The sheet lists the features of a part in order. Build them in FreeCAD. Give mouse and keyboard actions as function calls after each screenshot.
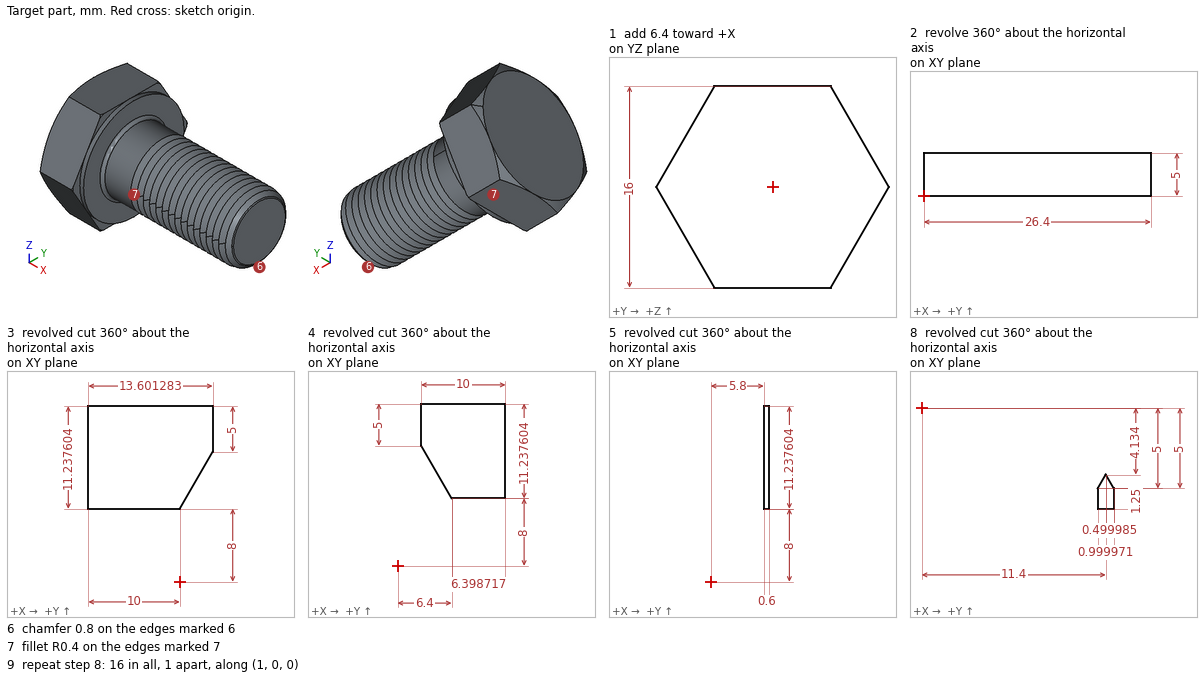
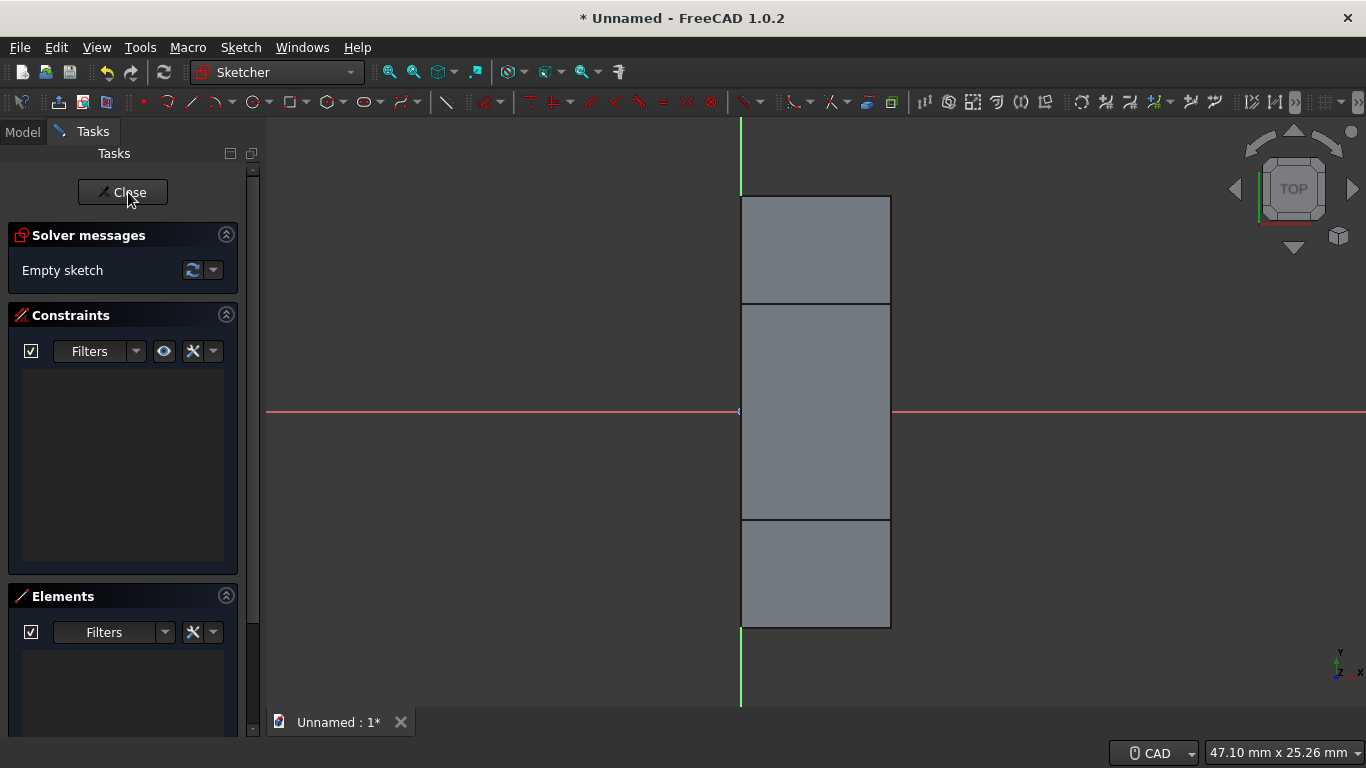
key(q)
key(s)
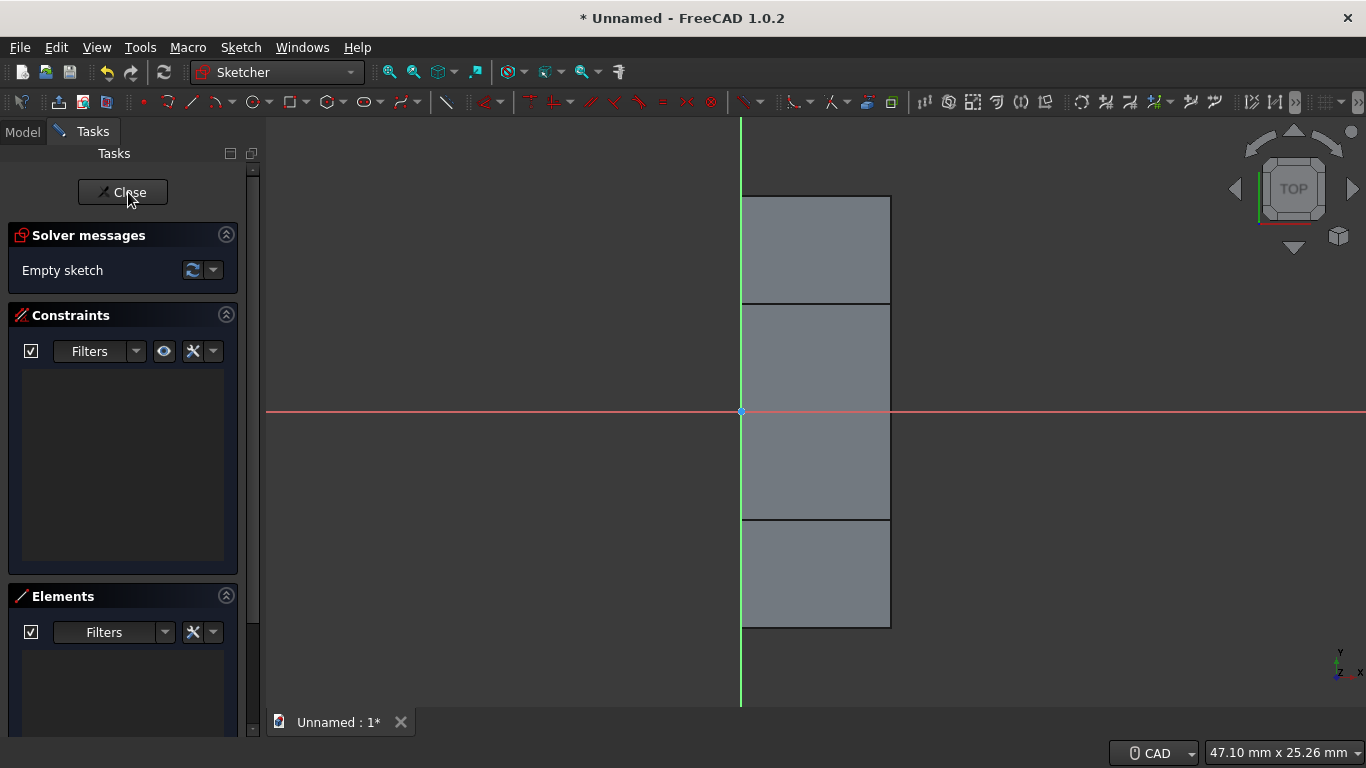
scroll(294, 676, down, 1)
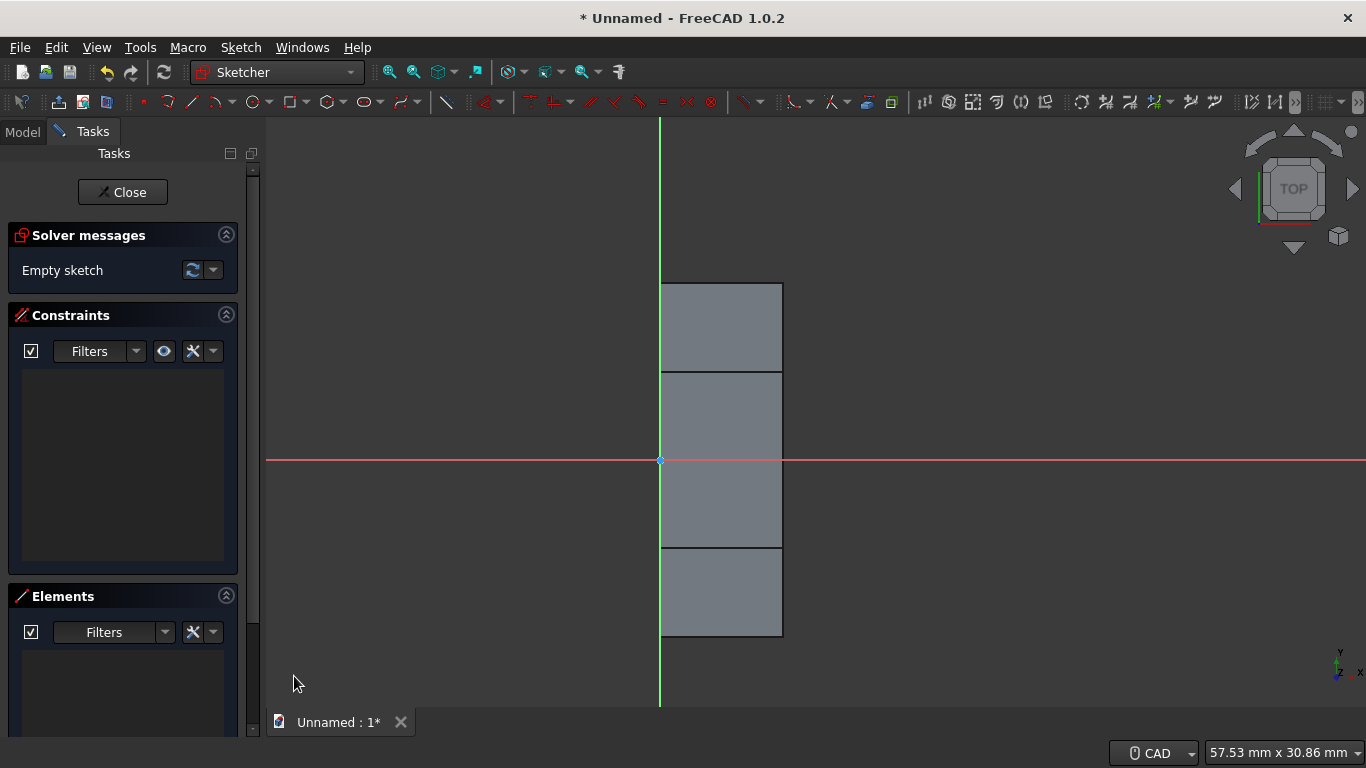
key(g)
key(r)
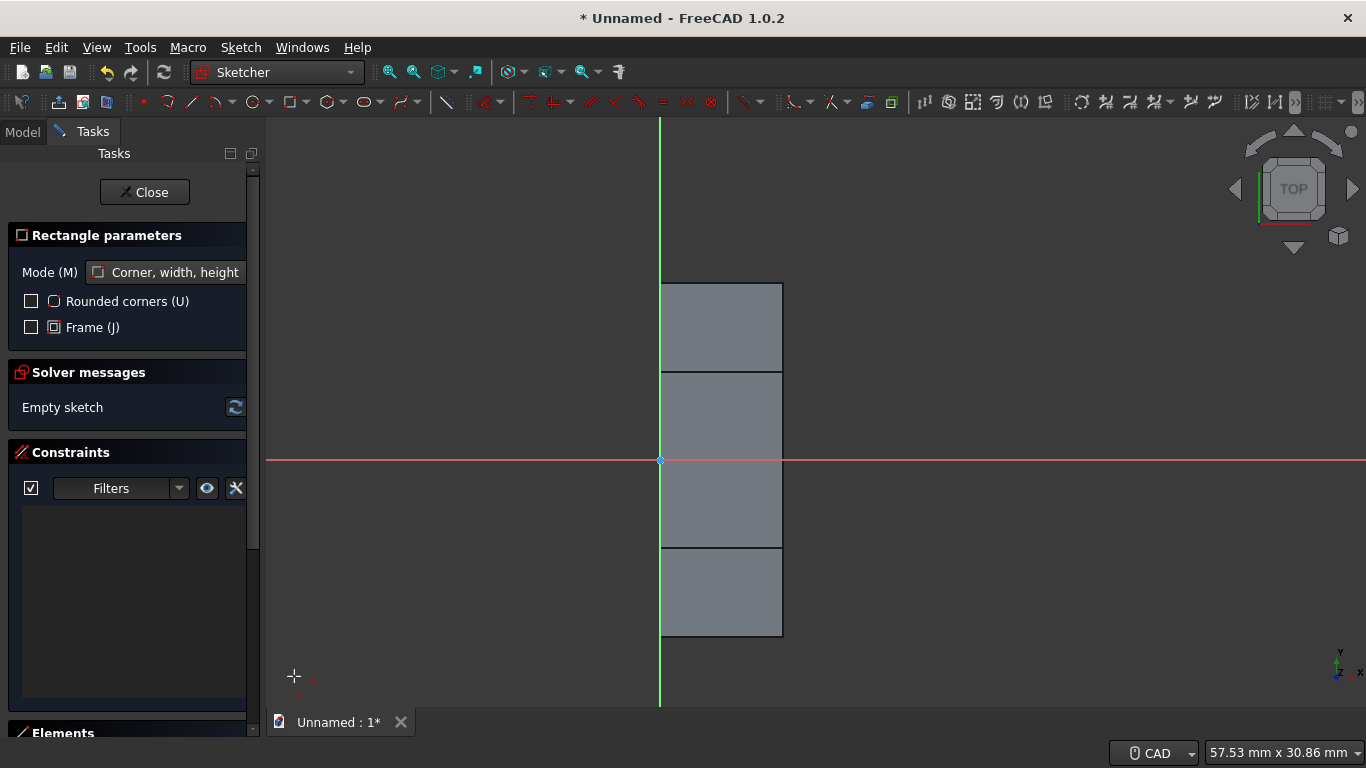
click(660, 460)
click(1165, 364)
key(Escape)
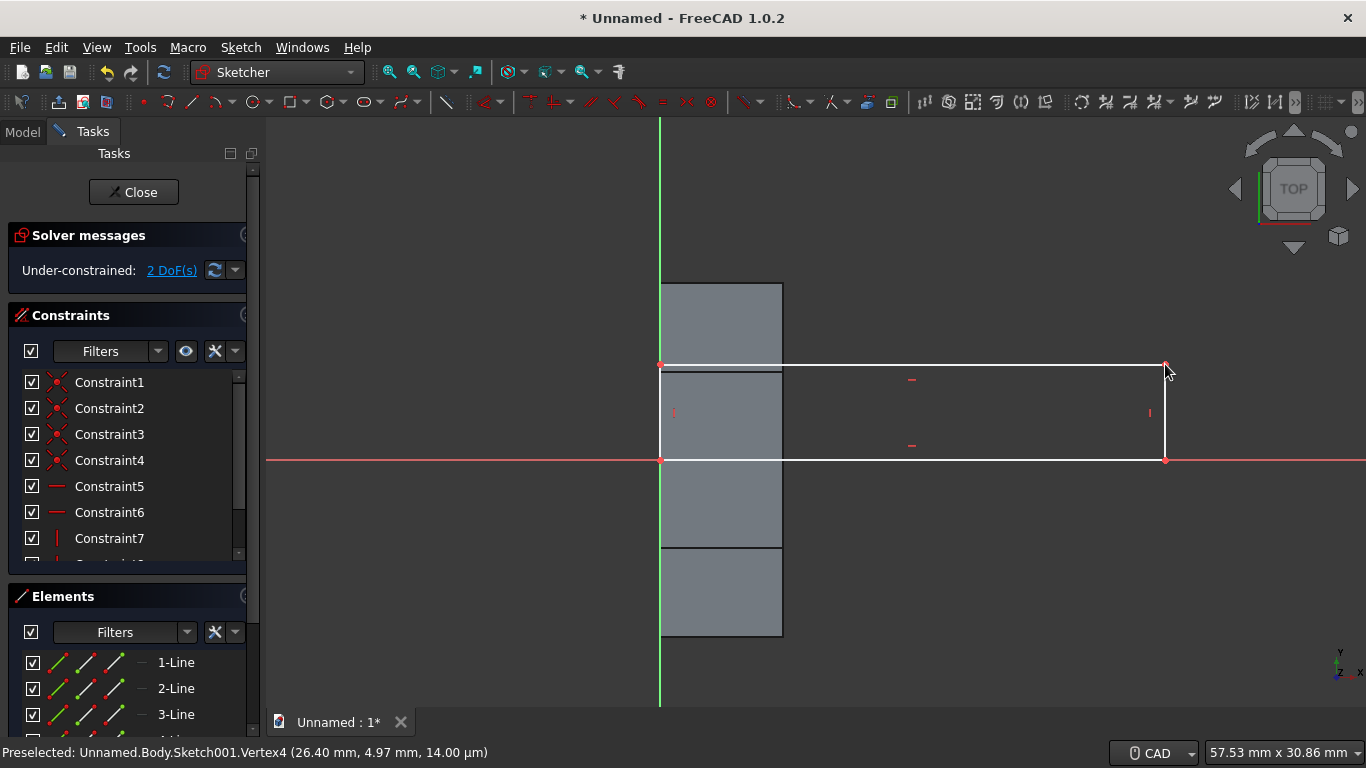
key(d)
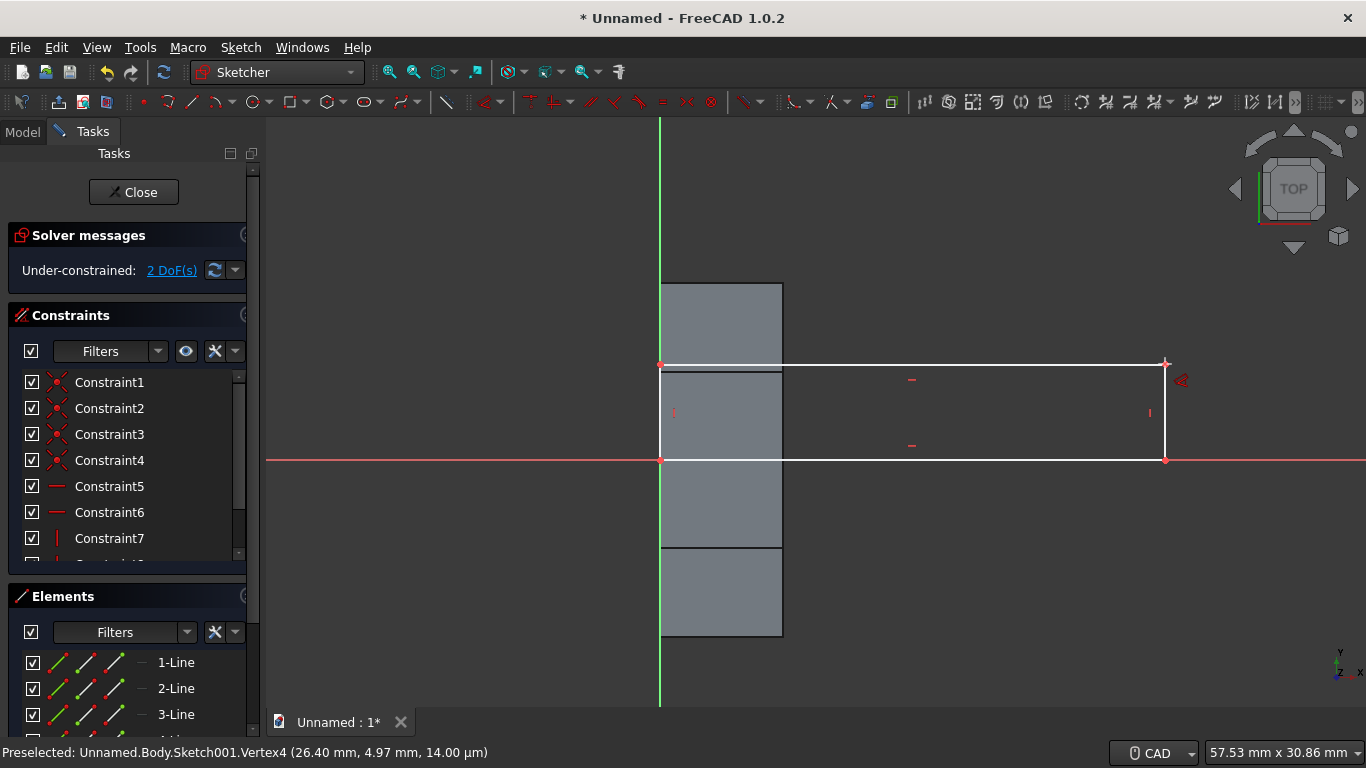
click(1165, 432)
click(1199, 413)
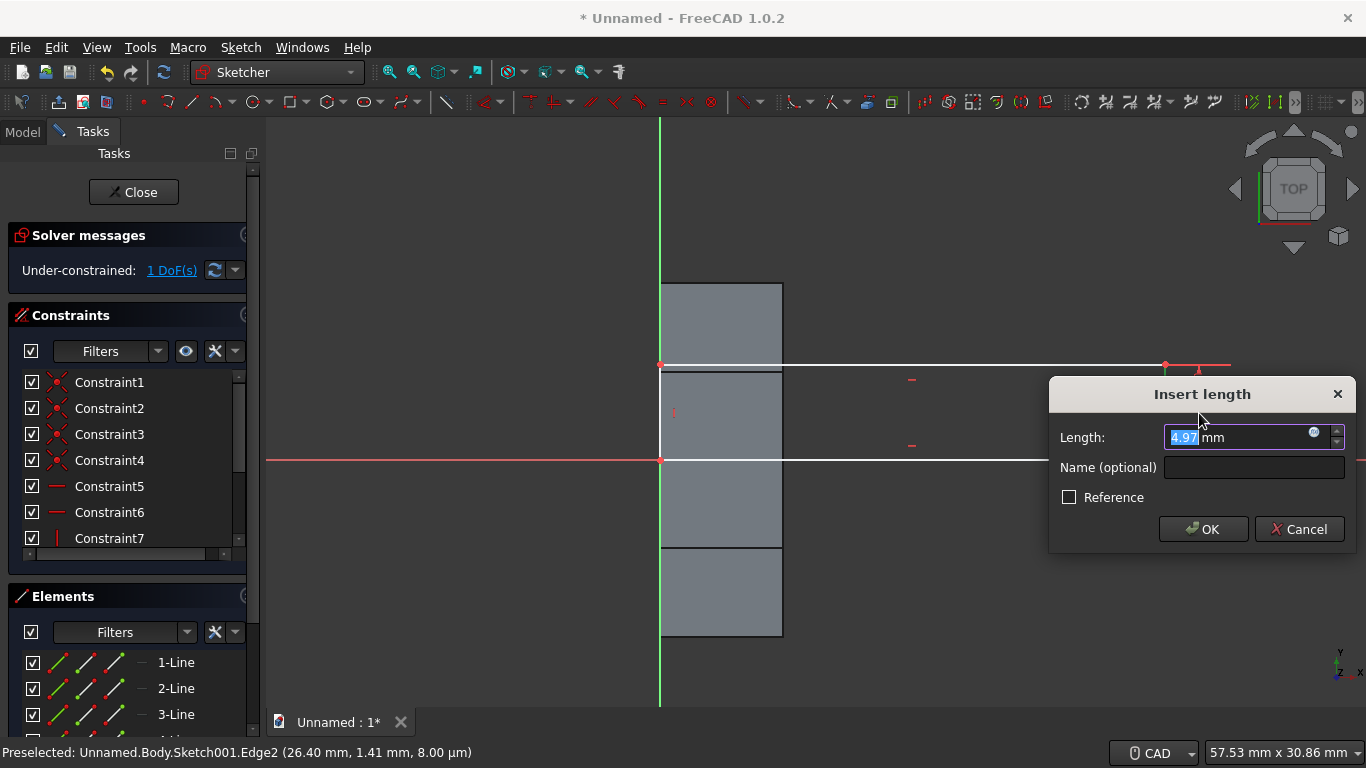
text(5)
key(Return)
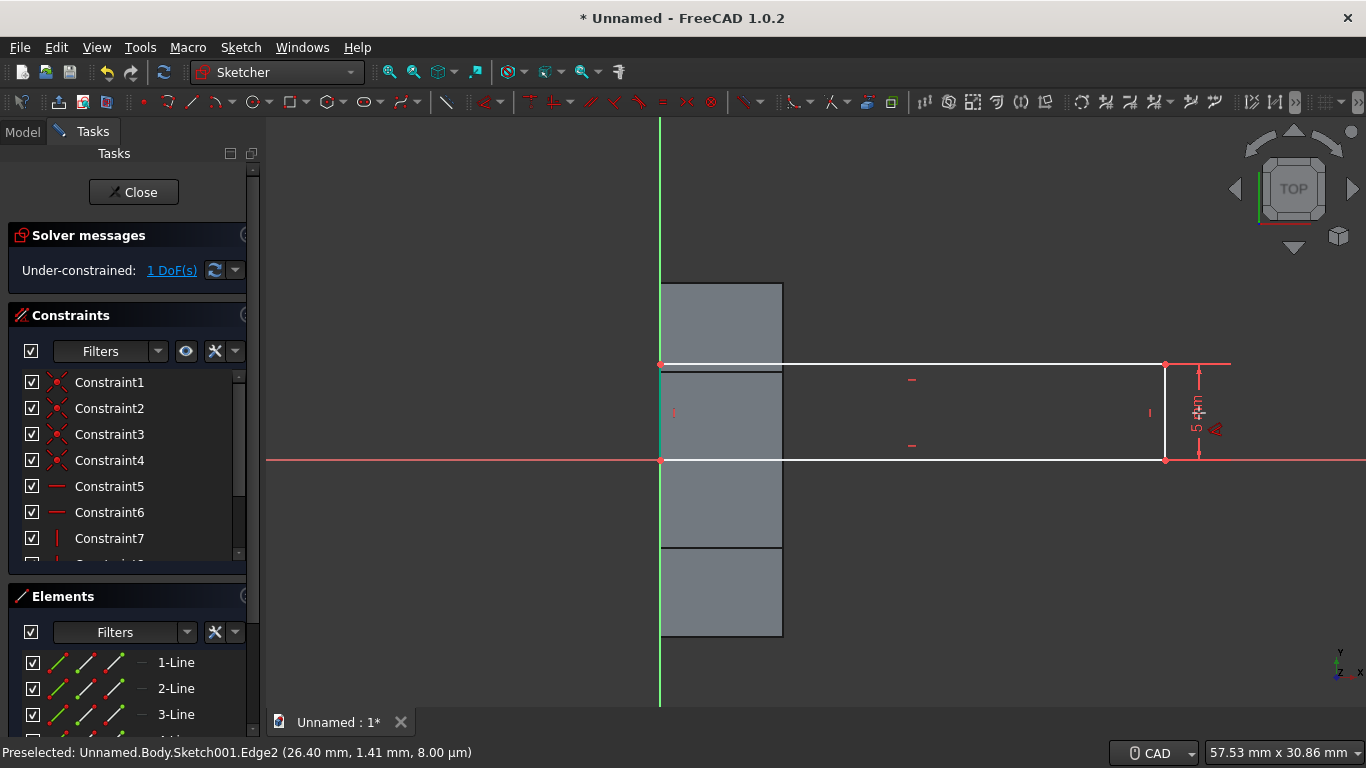
click(812, 460)
click(913, 494)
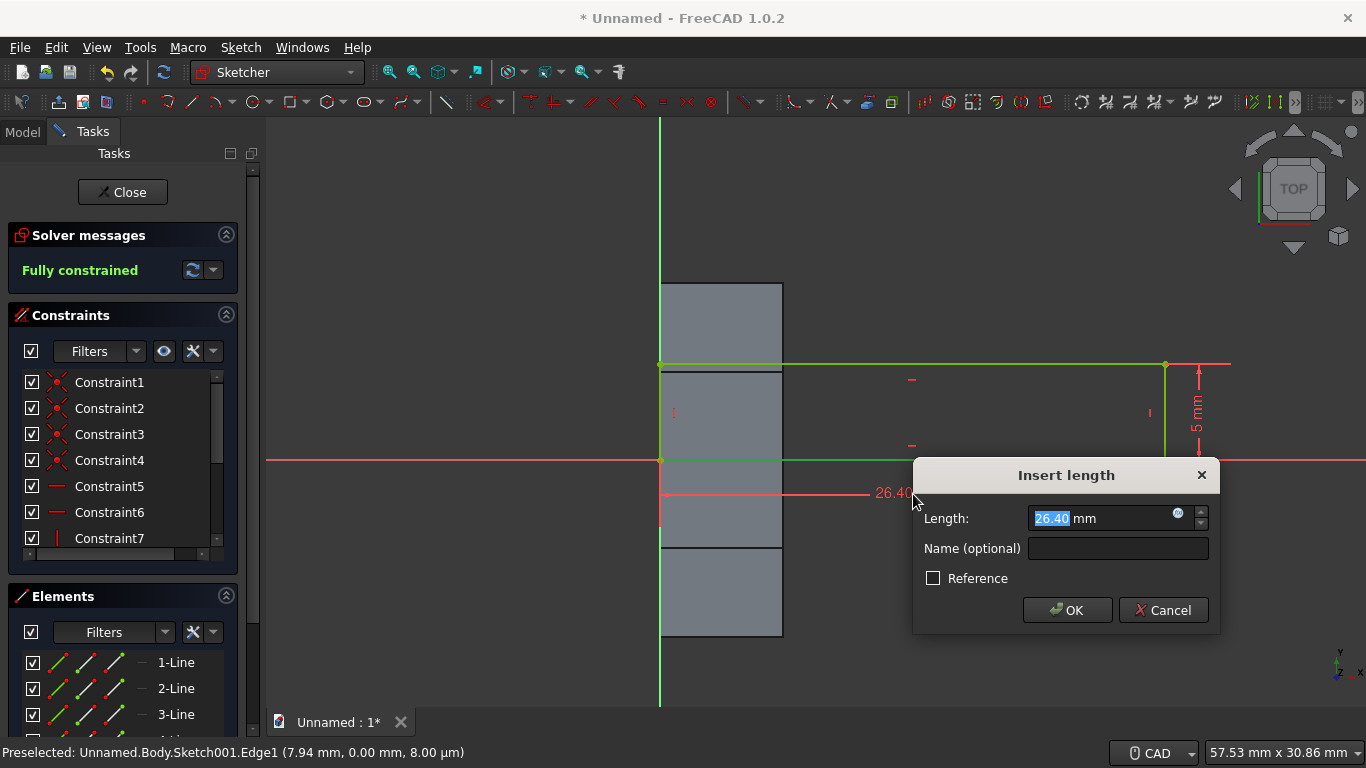
text(26.4)
key(Return)
key(Escape)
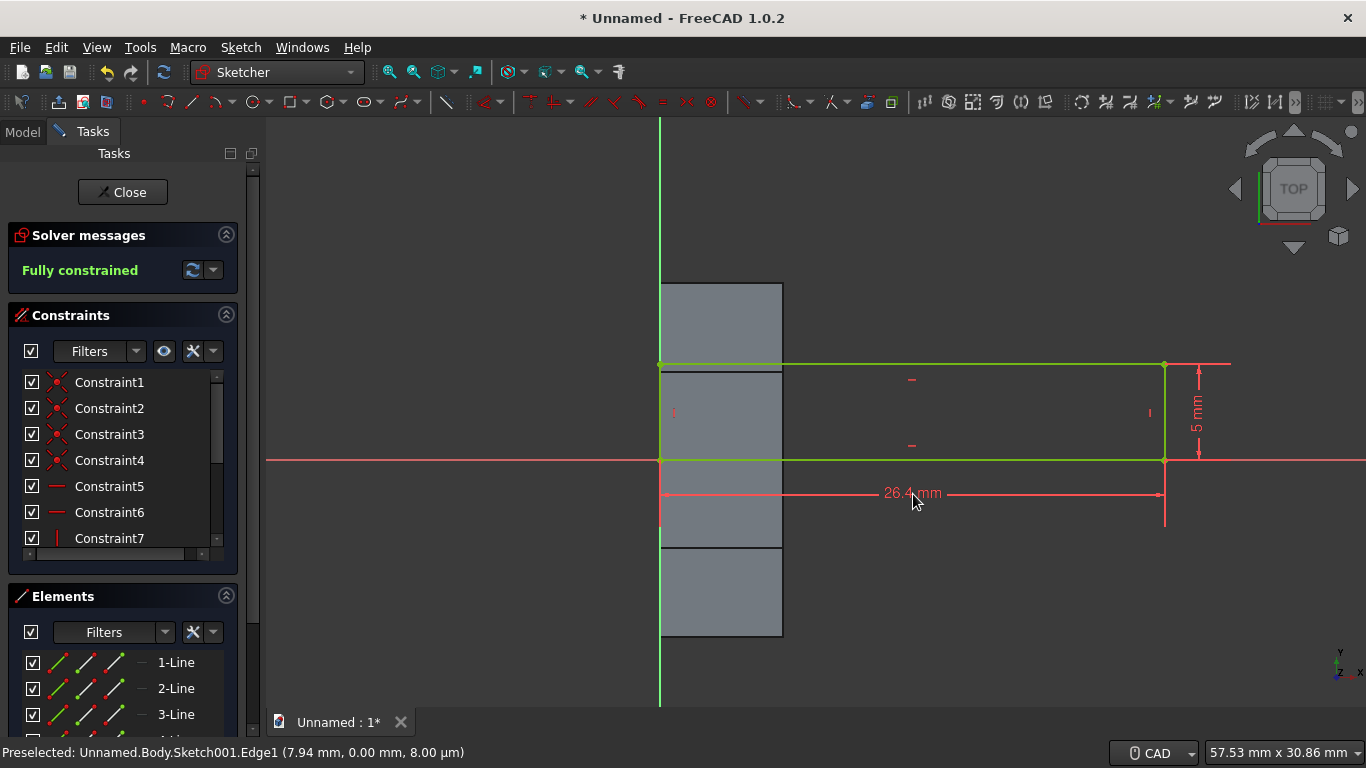
click(123, 192)